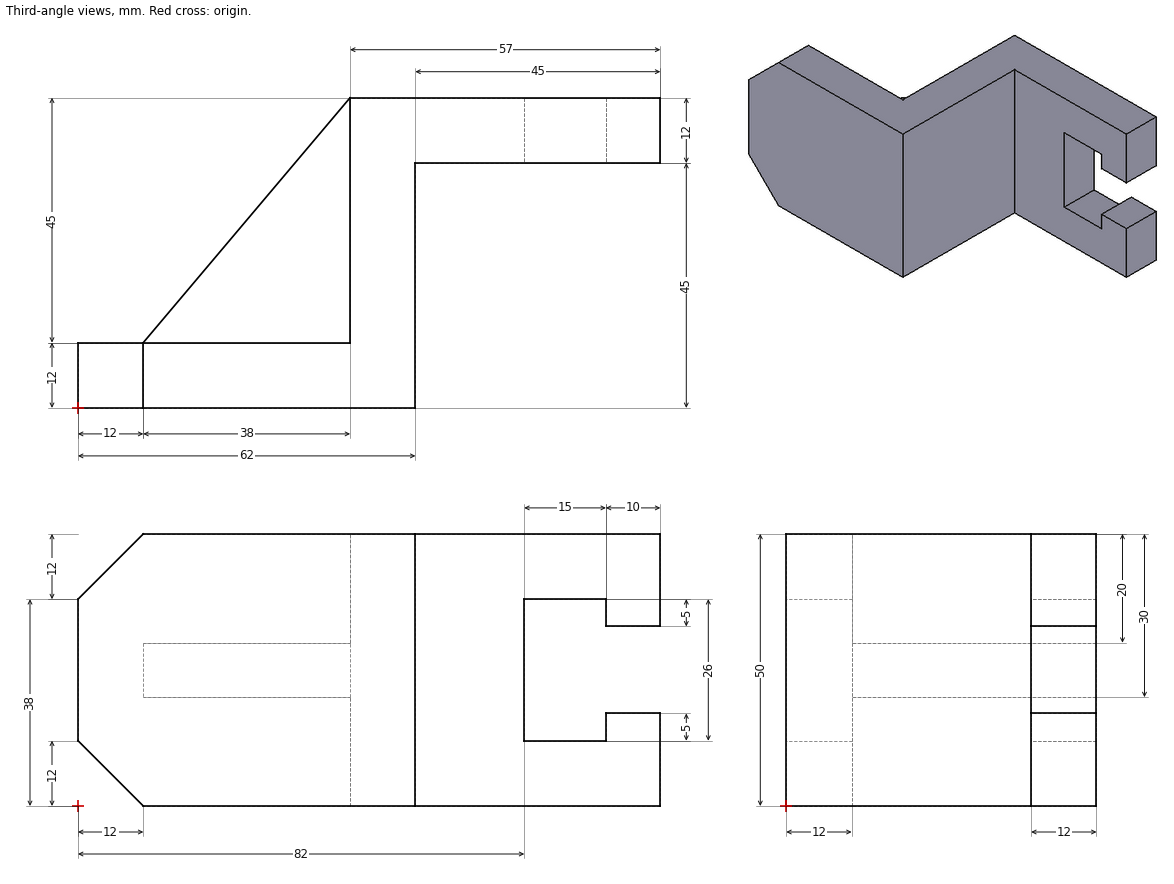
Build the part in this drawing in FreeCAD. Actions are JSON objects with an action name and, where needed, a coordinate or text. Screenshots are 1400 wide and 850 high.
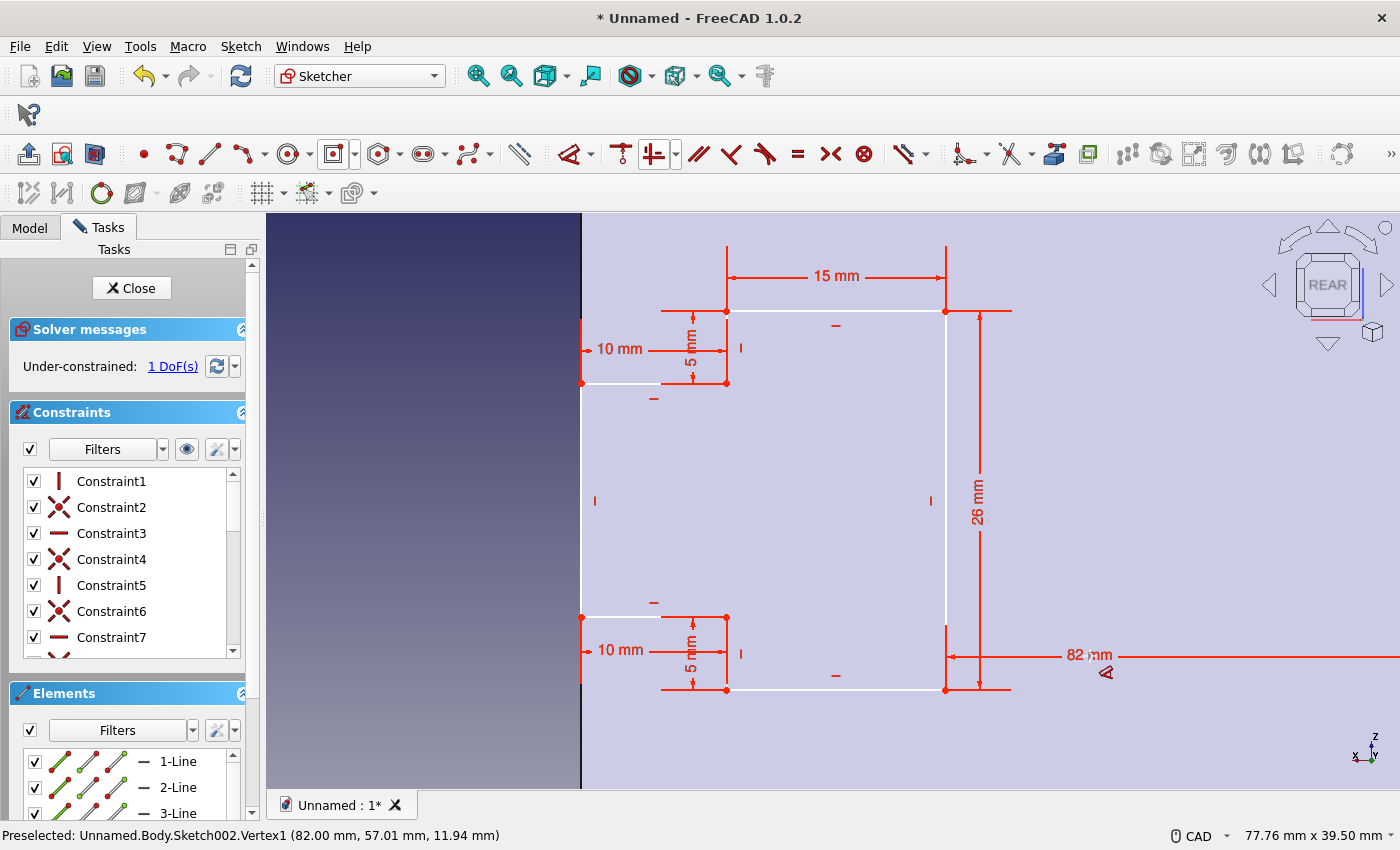
{"action": "left_click", "coordinate": [946, 690]}
{"action": "left_click", "coordinate": [912, 726]}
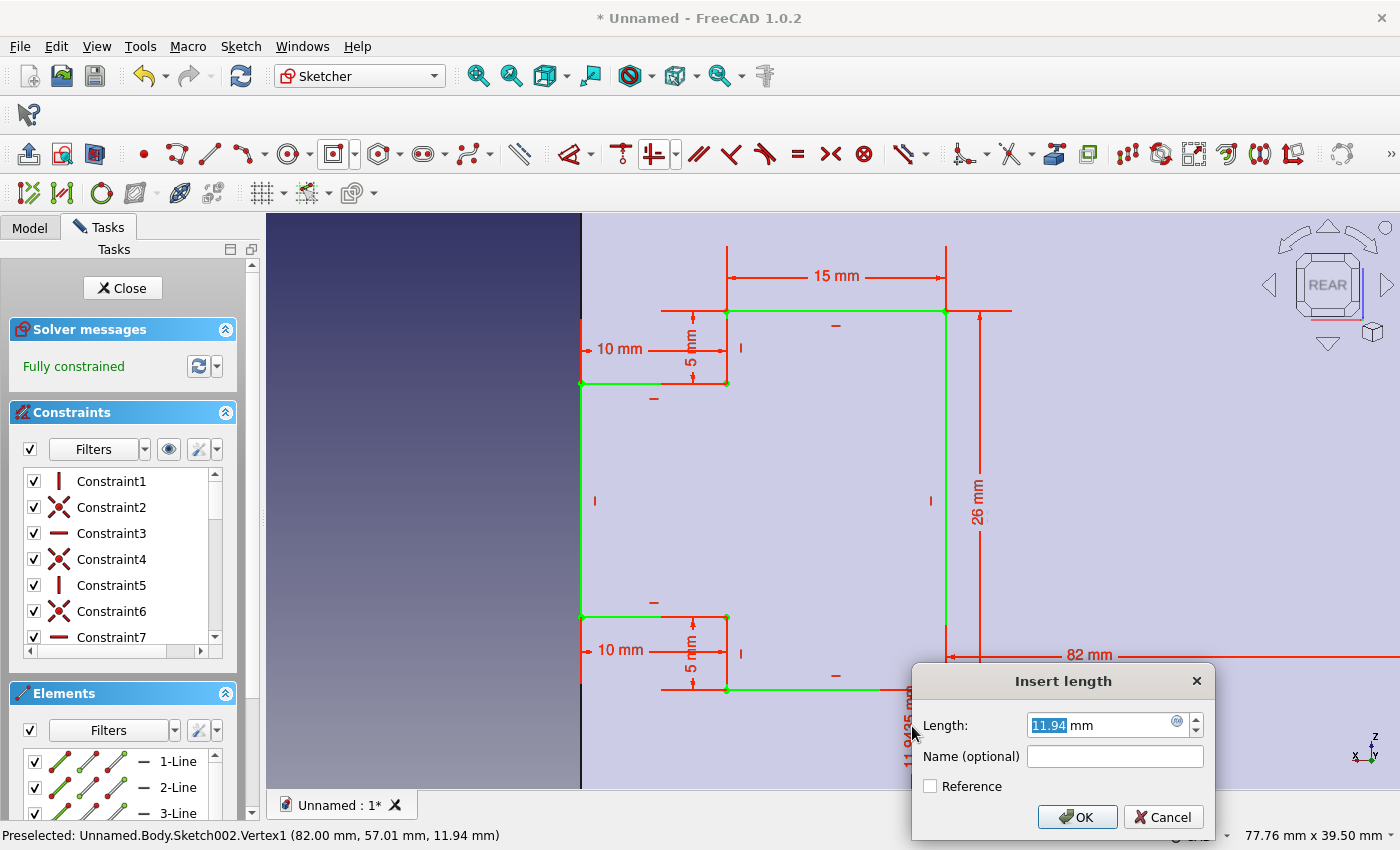
{"action": "type", "text": "12"}
{"action": "key", "text": "Return"}
{"action": "key", "text": "Escape"}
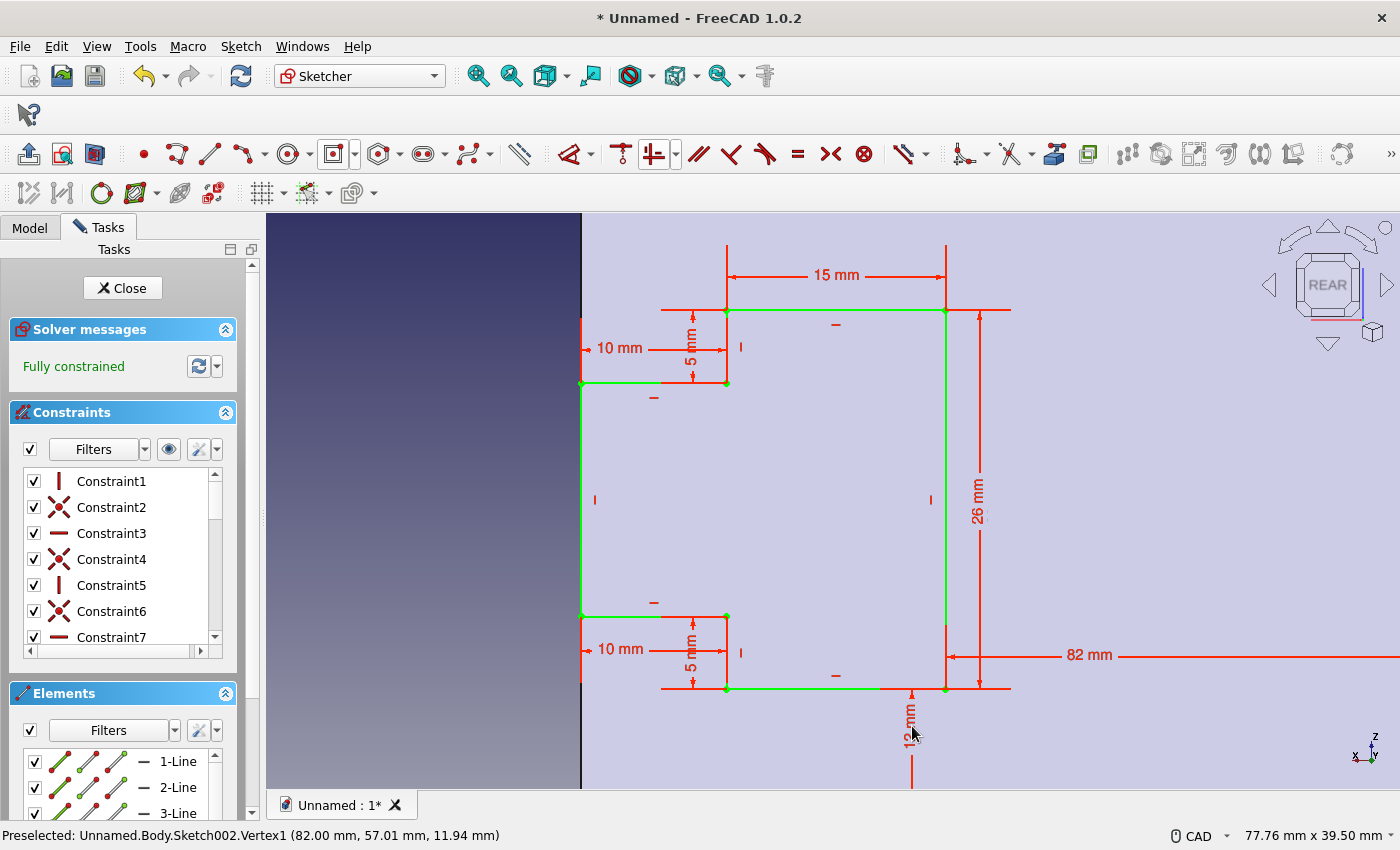
{"action": "left_click", "coordinate": [123, 288]}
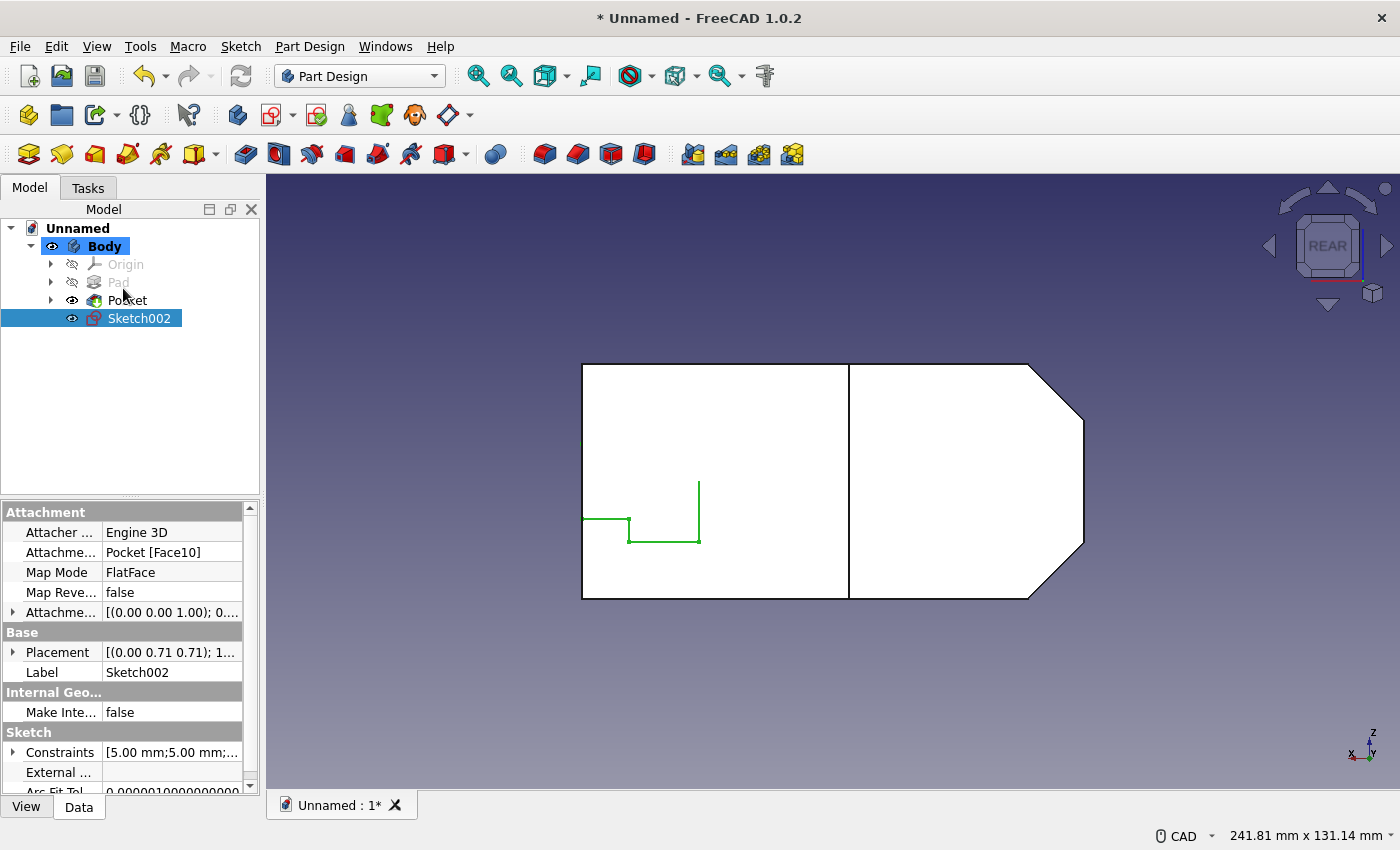
{"action": "left_click", "coordinate": [246, 154]}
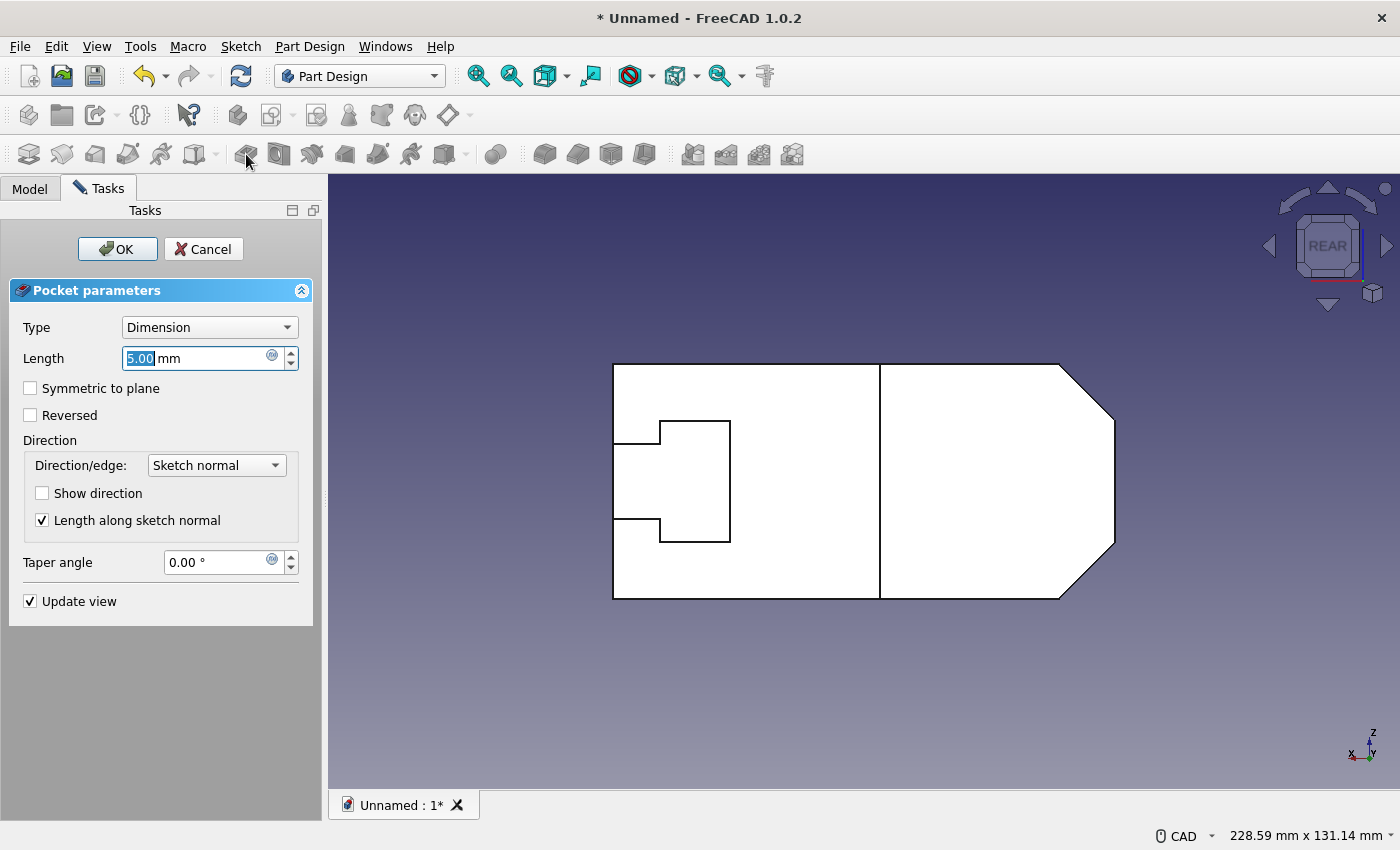
{"action": "type", "text": "12"}
{"action": "key", "text": "Tab"}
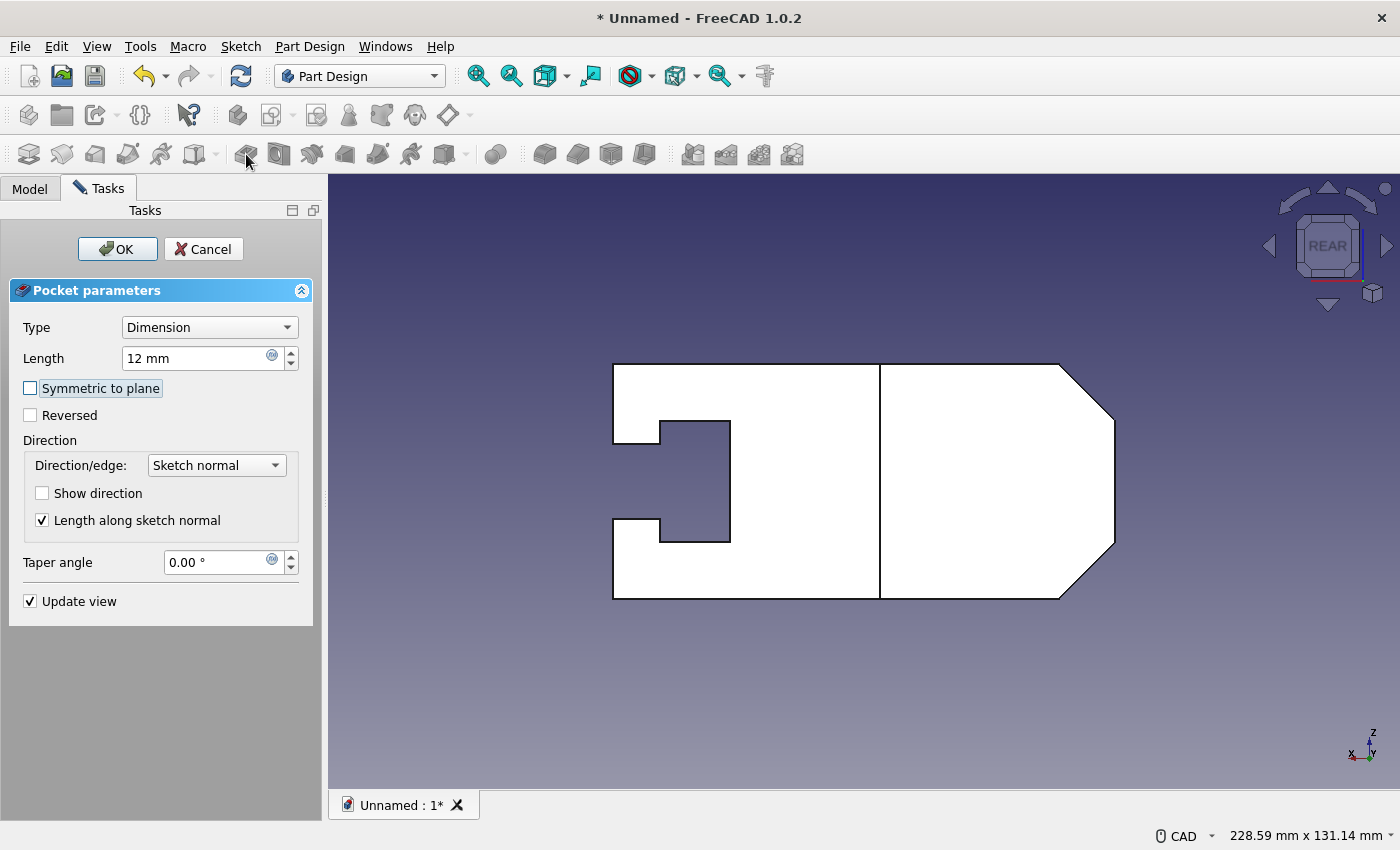
{"action": "left_click", "coordinate": [118, 249]}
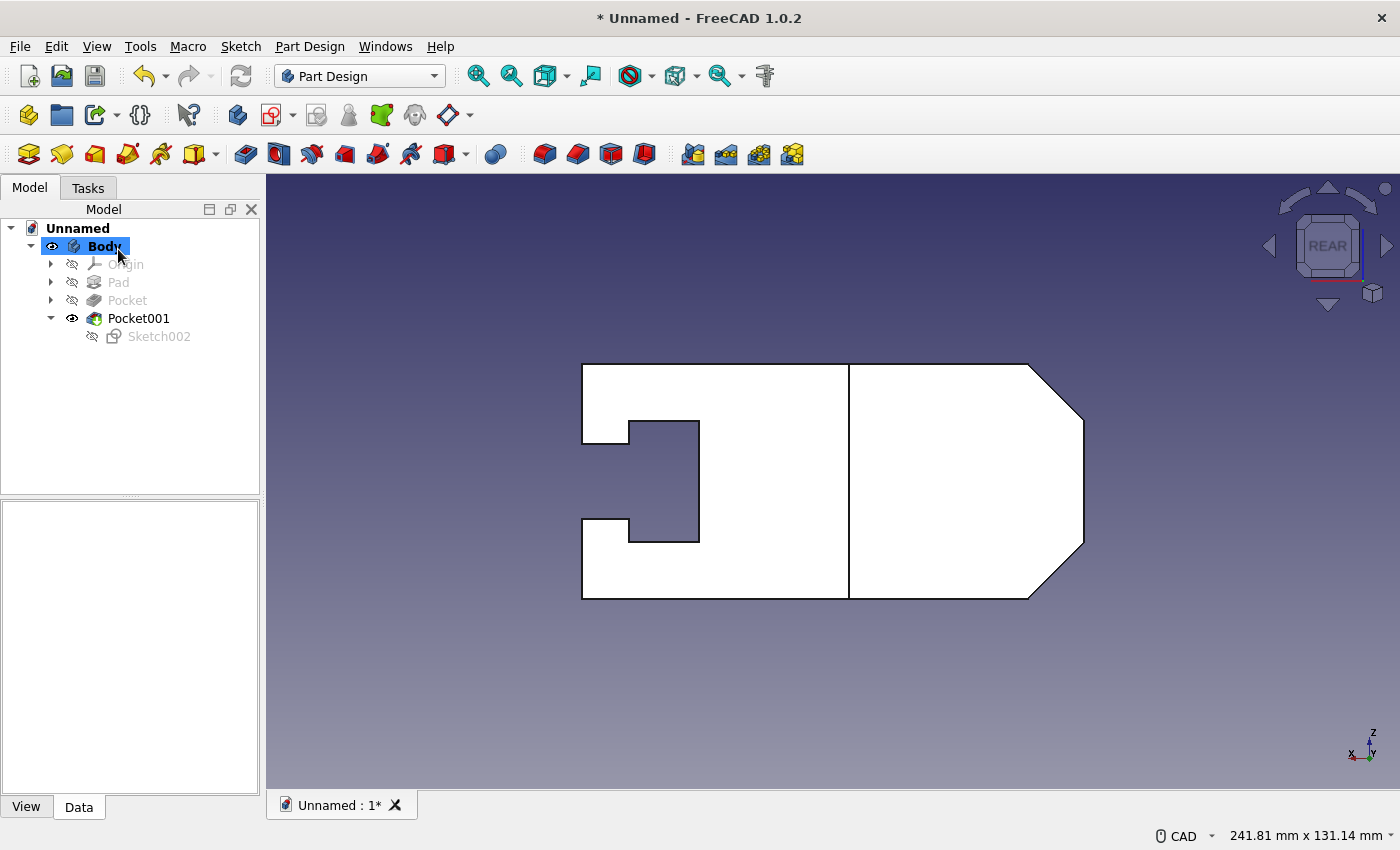
{"action": "left_click", "coordinate": [479, 76]}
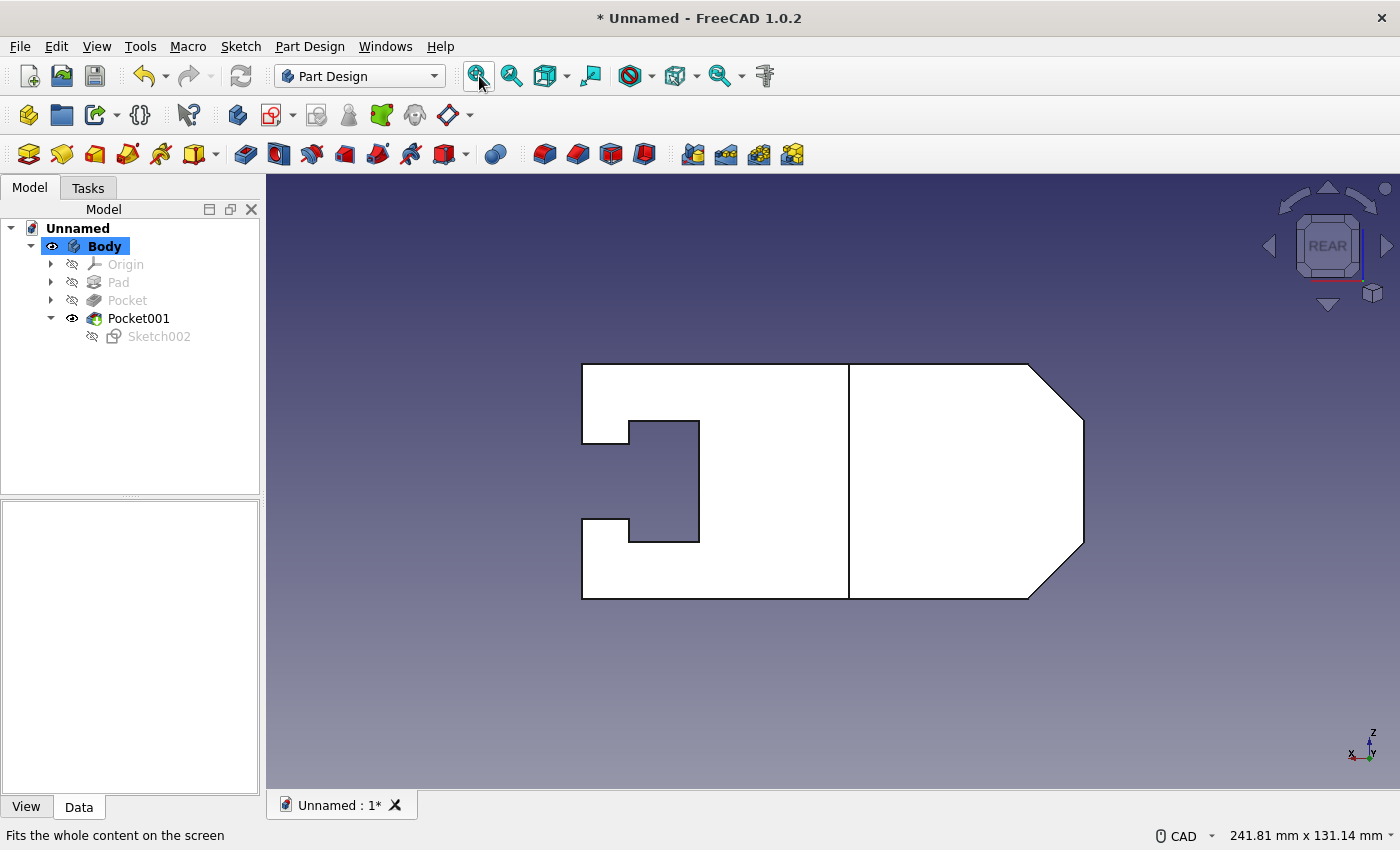
{"action": "key", "text": "0"}